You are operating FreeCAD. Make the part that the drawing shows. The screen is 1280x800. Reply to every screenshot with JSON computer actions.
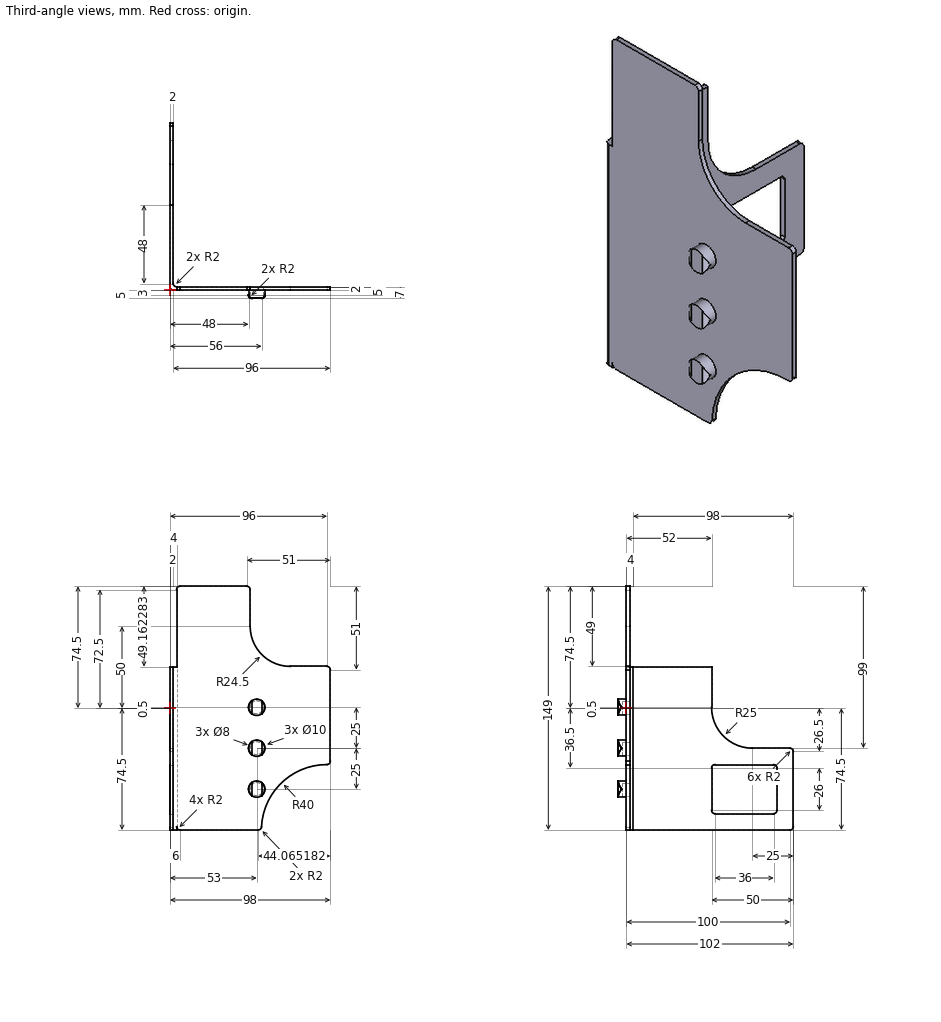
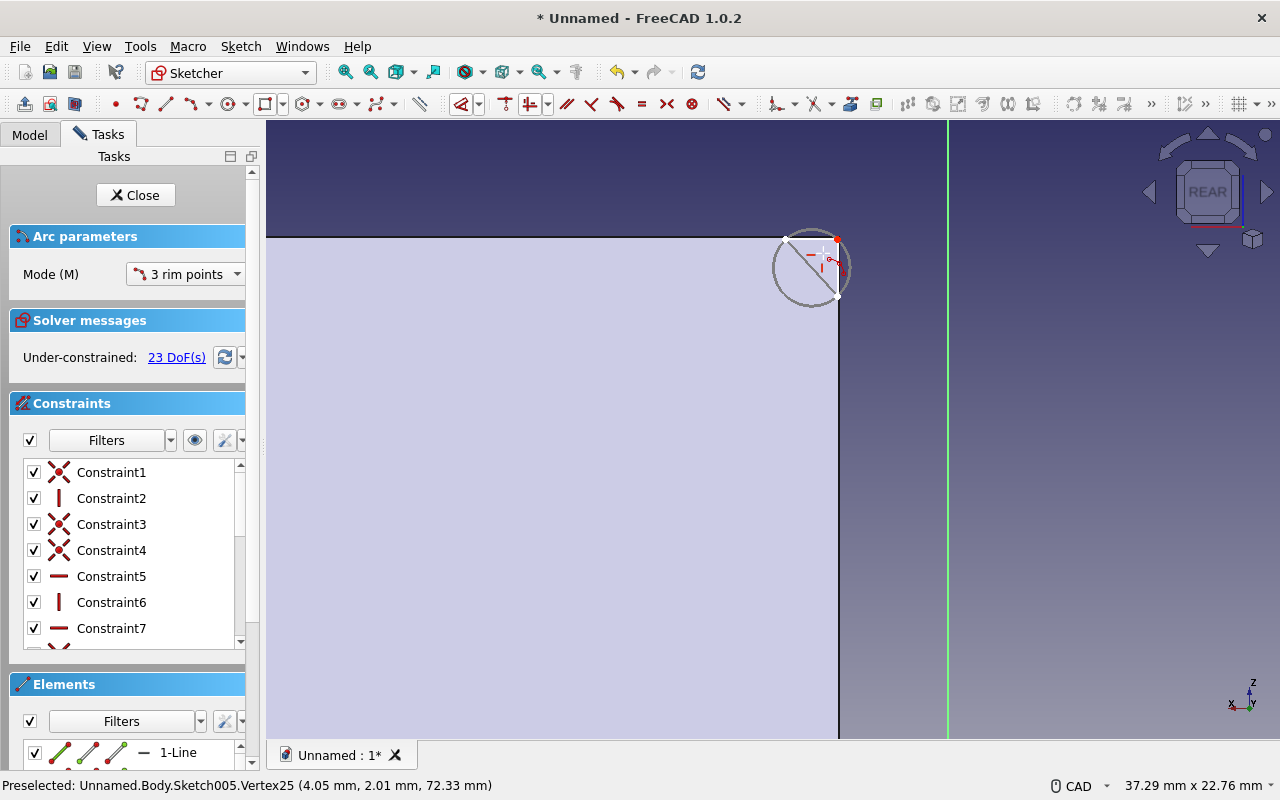
{"action": "left_click", "coordinate": [823, 253]}
{"action": "key", "text": "Escape"}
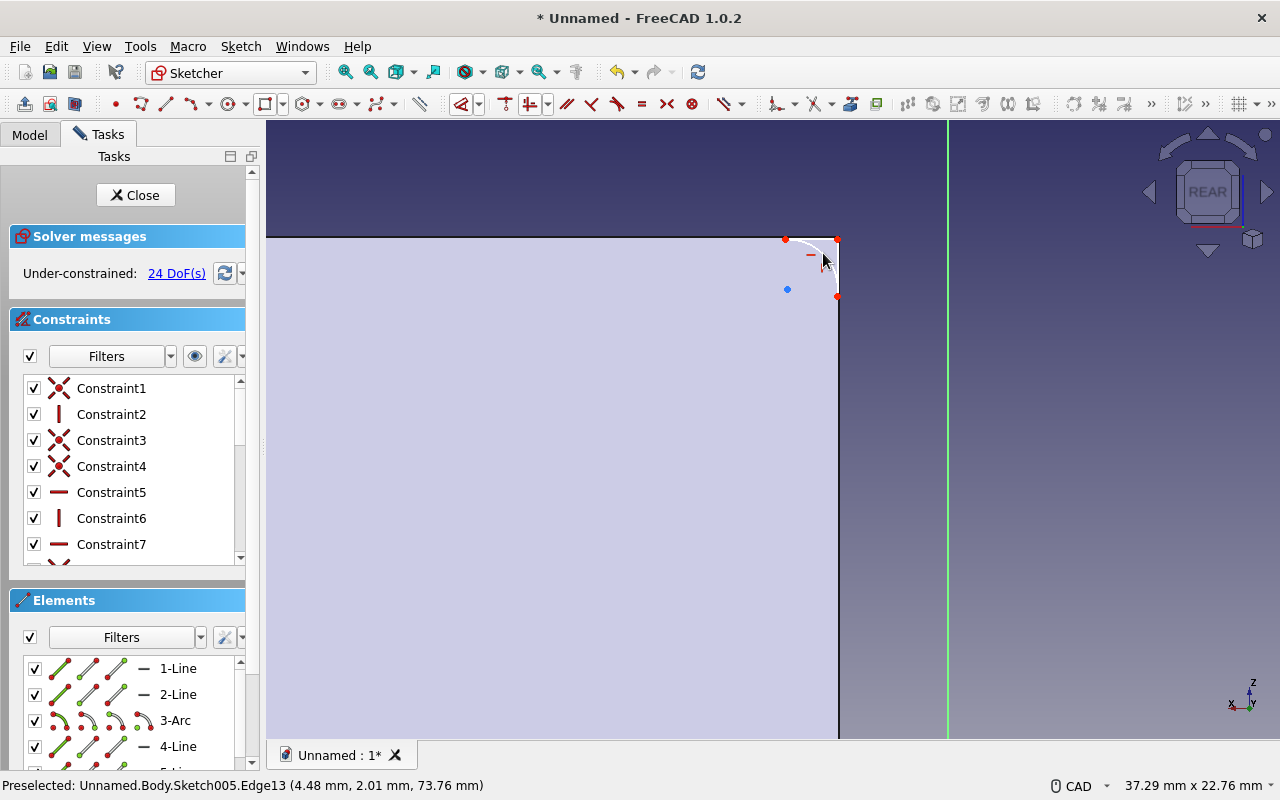
{"action": "scroll", "coordinate": [813, 247], "scroll_direction": "down", "scroll_amount": 12}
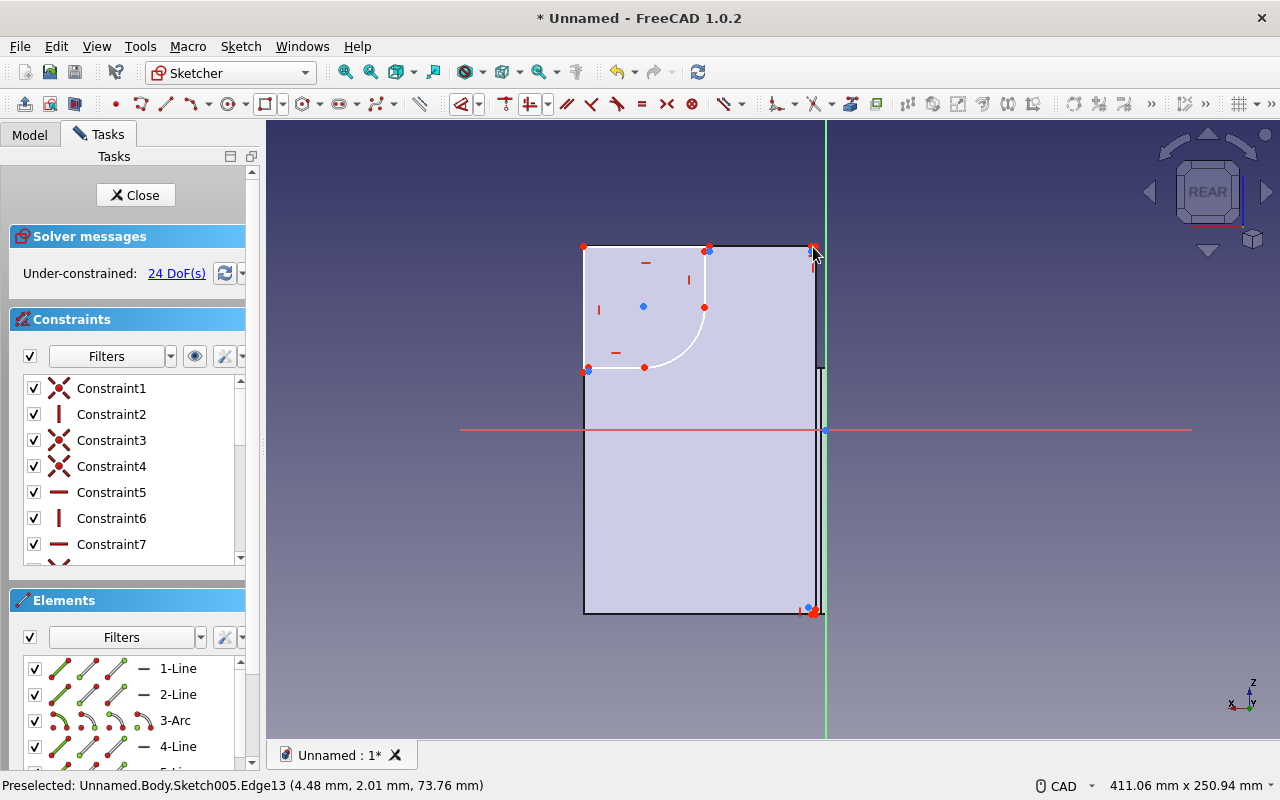
{"action": "scroll", "coordinate": [815, 614], "scroll_direction": "up", "scroll_amount": 12}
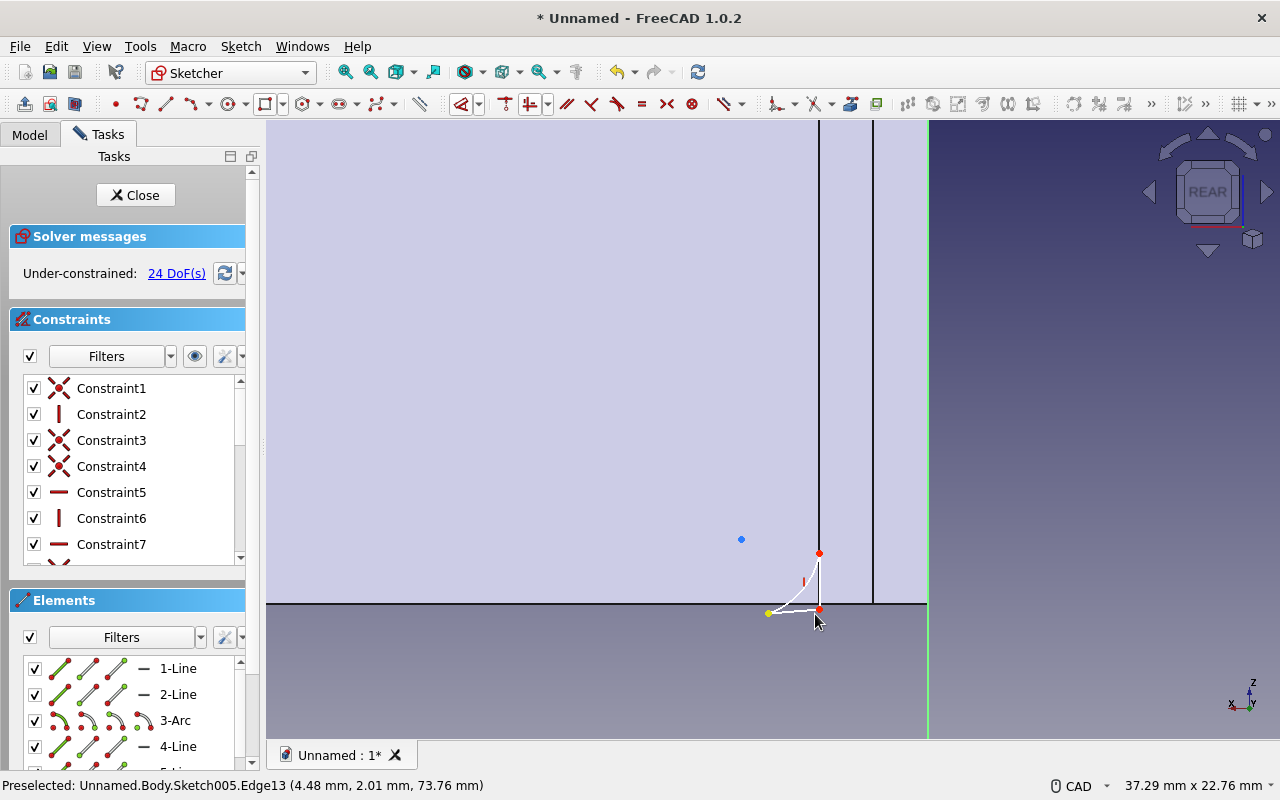
{"action": "left_click", "coordinate": [804, 611]}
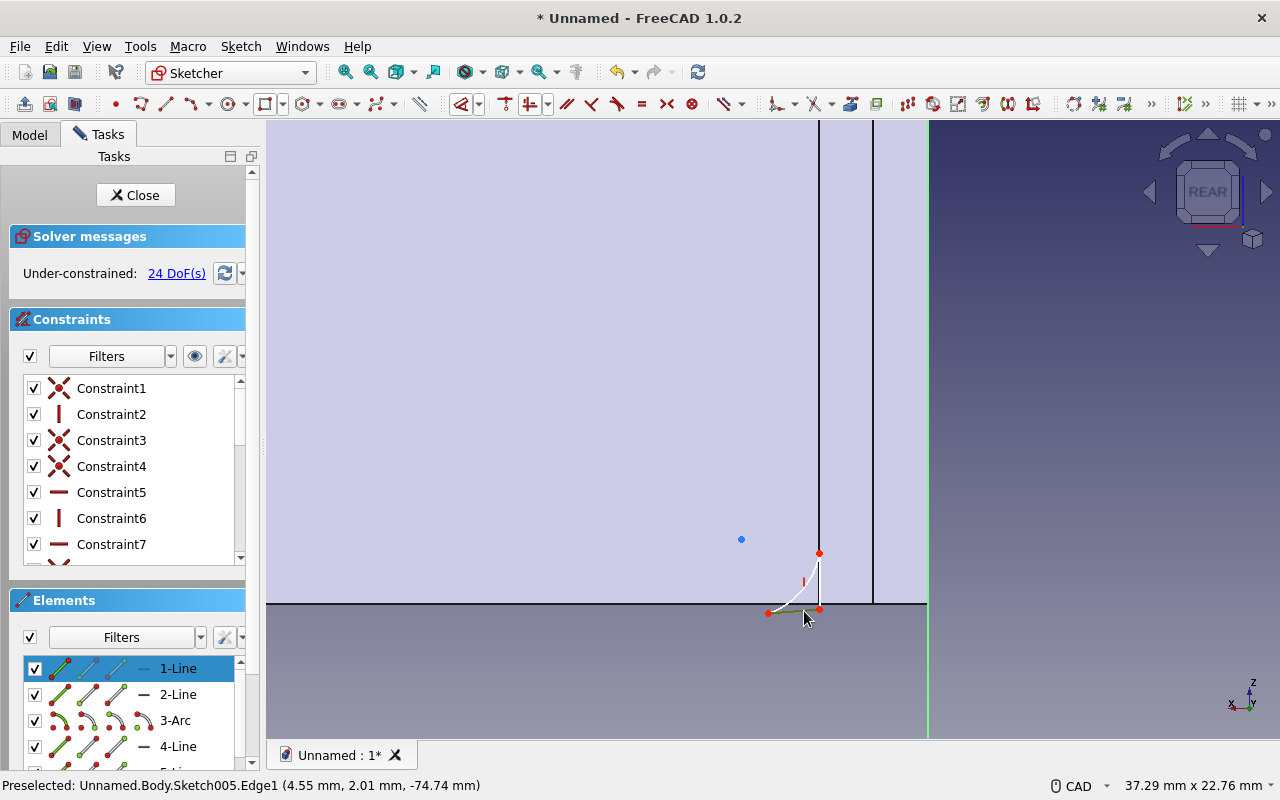
{"action": "scroll", "coordinate": [790, 602], "scroll_direction": "up", "scroll_amount": 2}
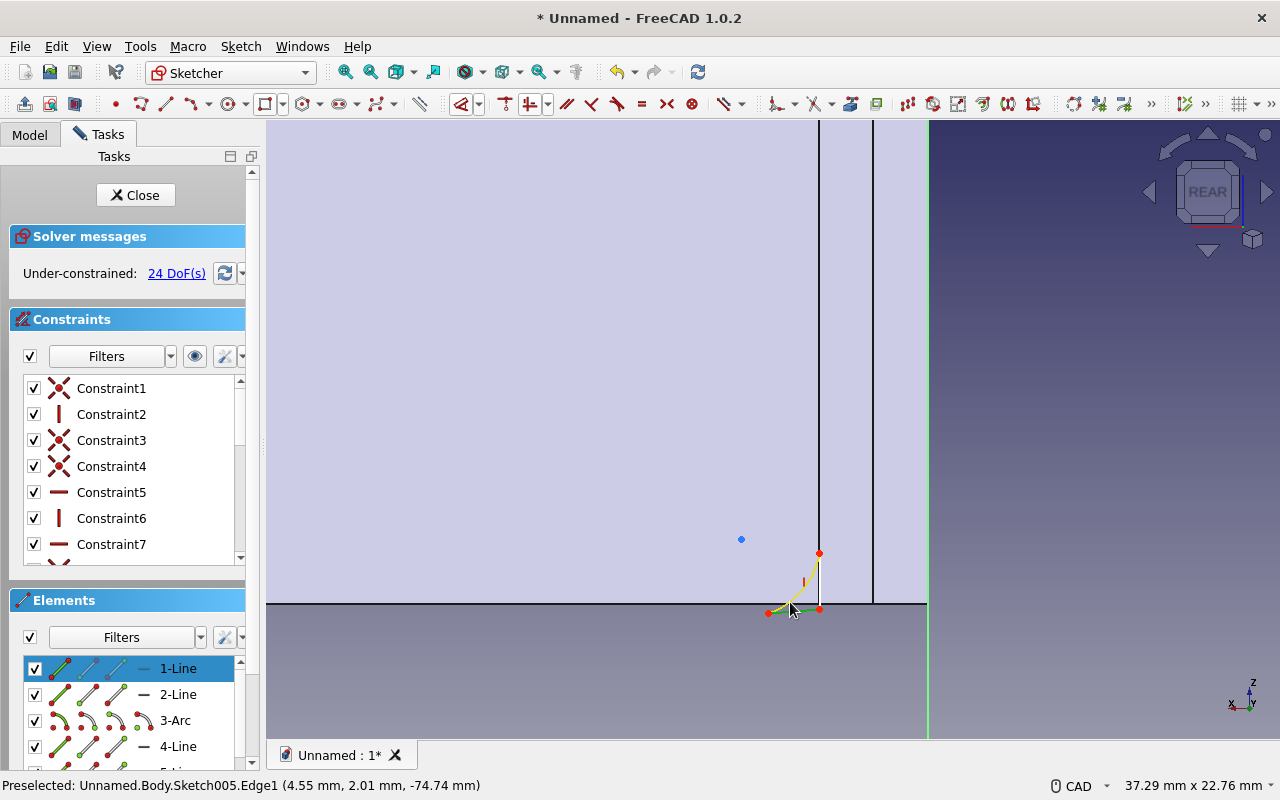
{"action": "left_click", "coordinate": [790, 601]}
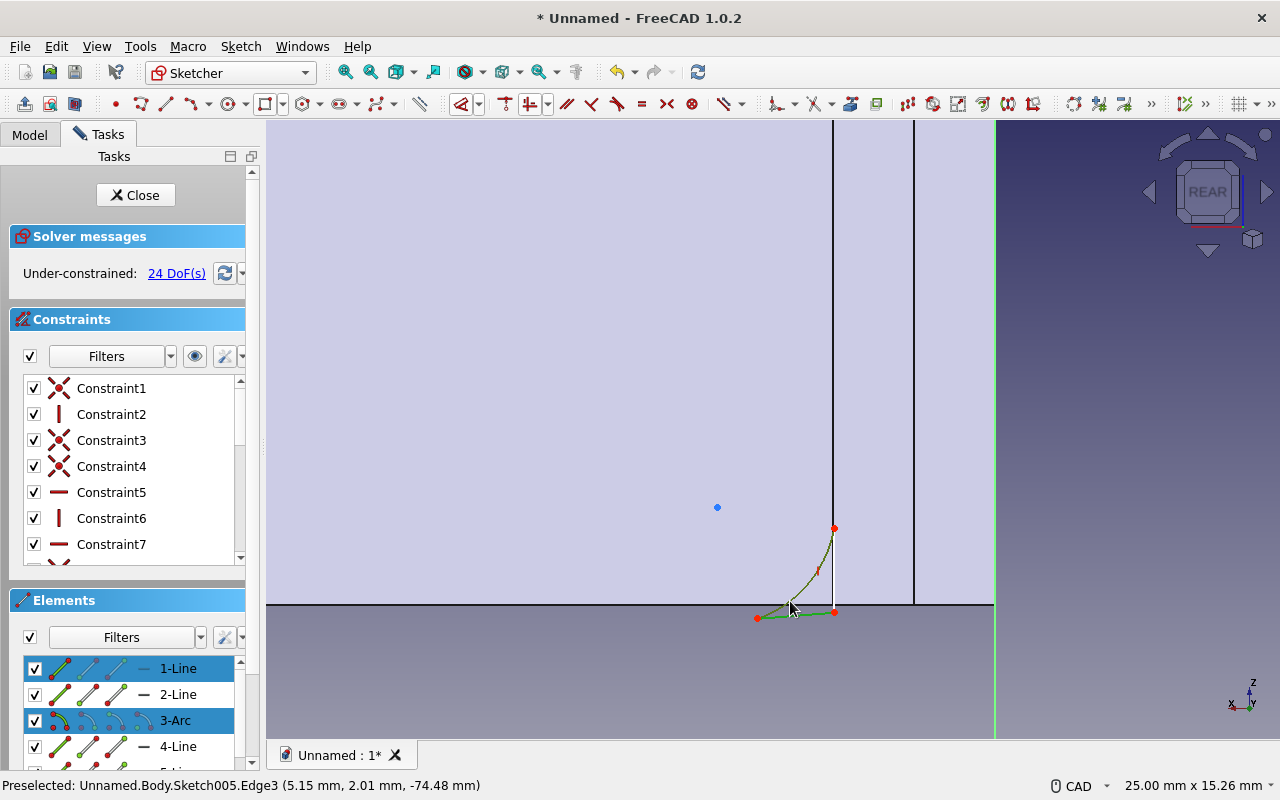
{"action": "key", "text": "t"}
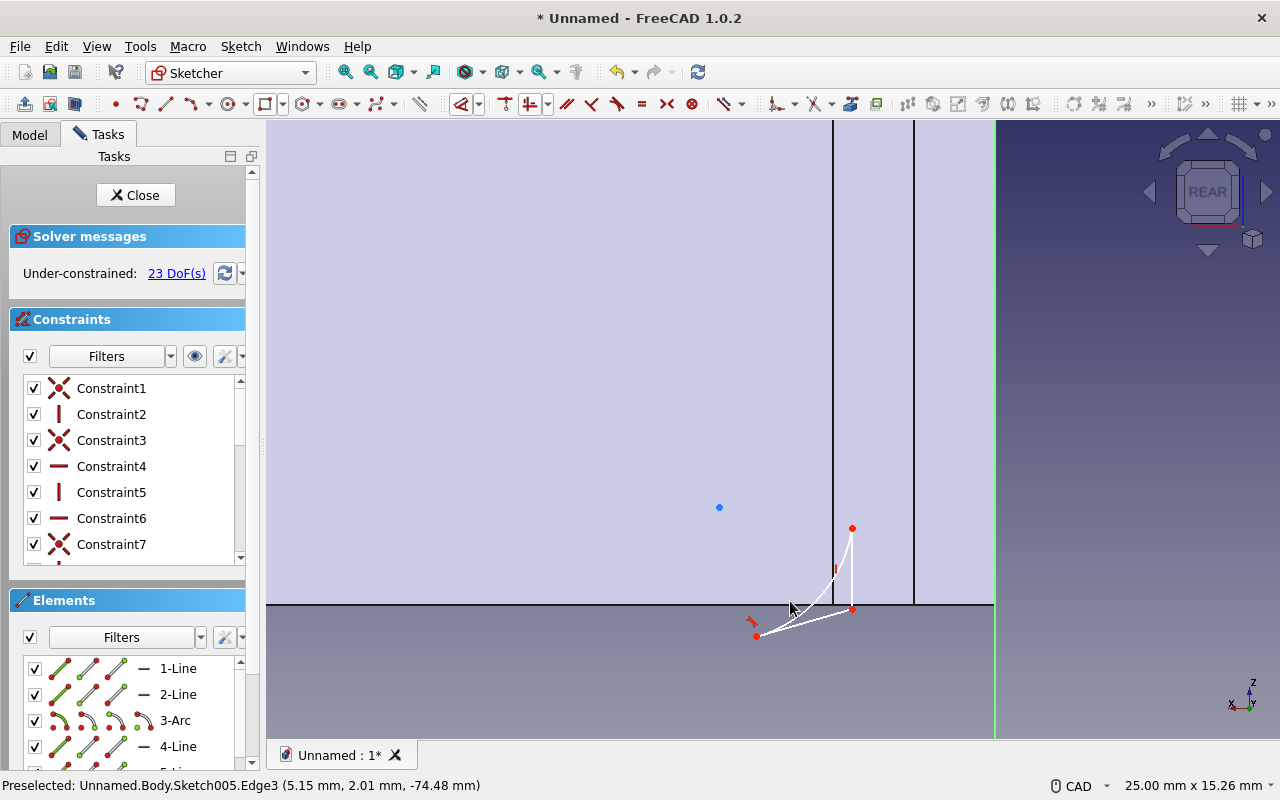
{"action": "left_click", "coordinate": [852, 585]}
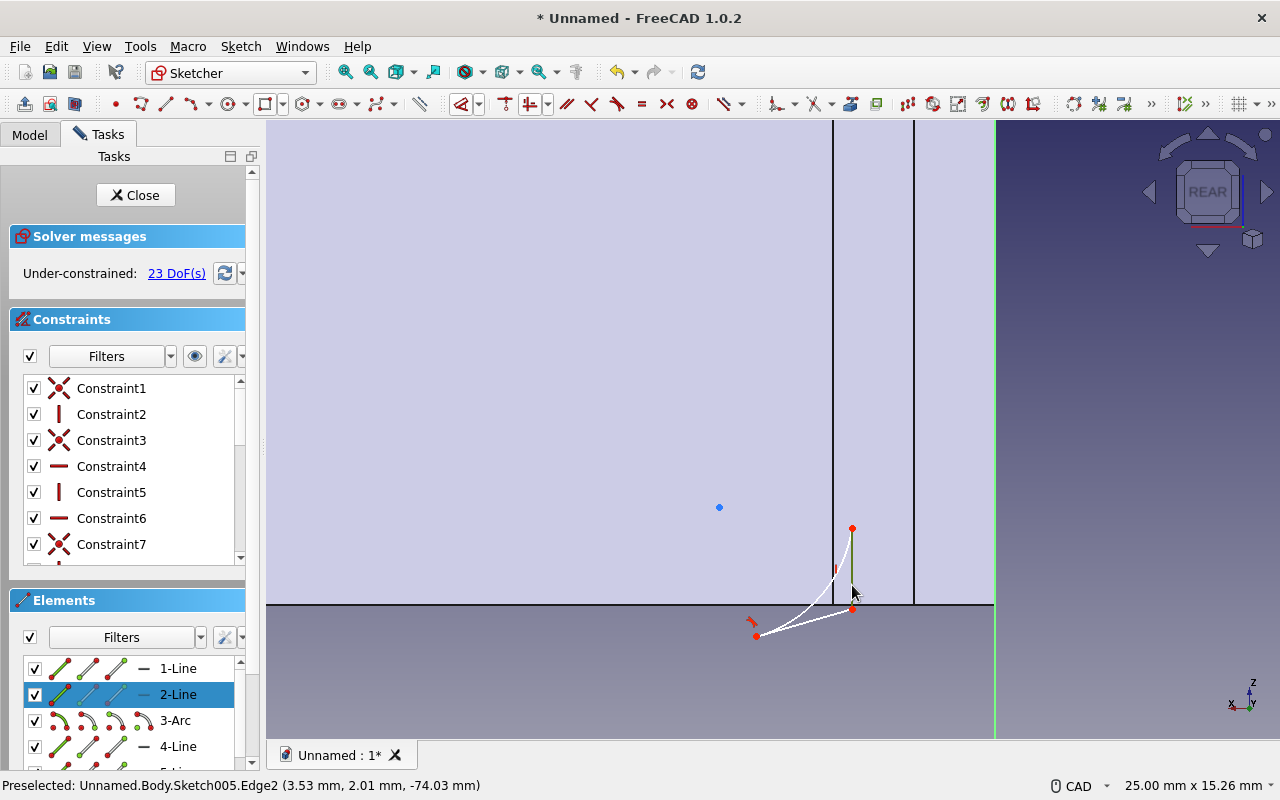
{"action": "left_click", "coordinate": [820, 597]}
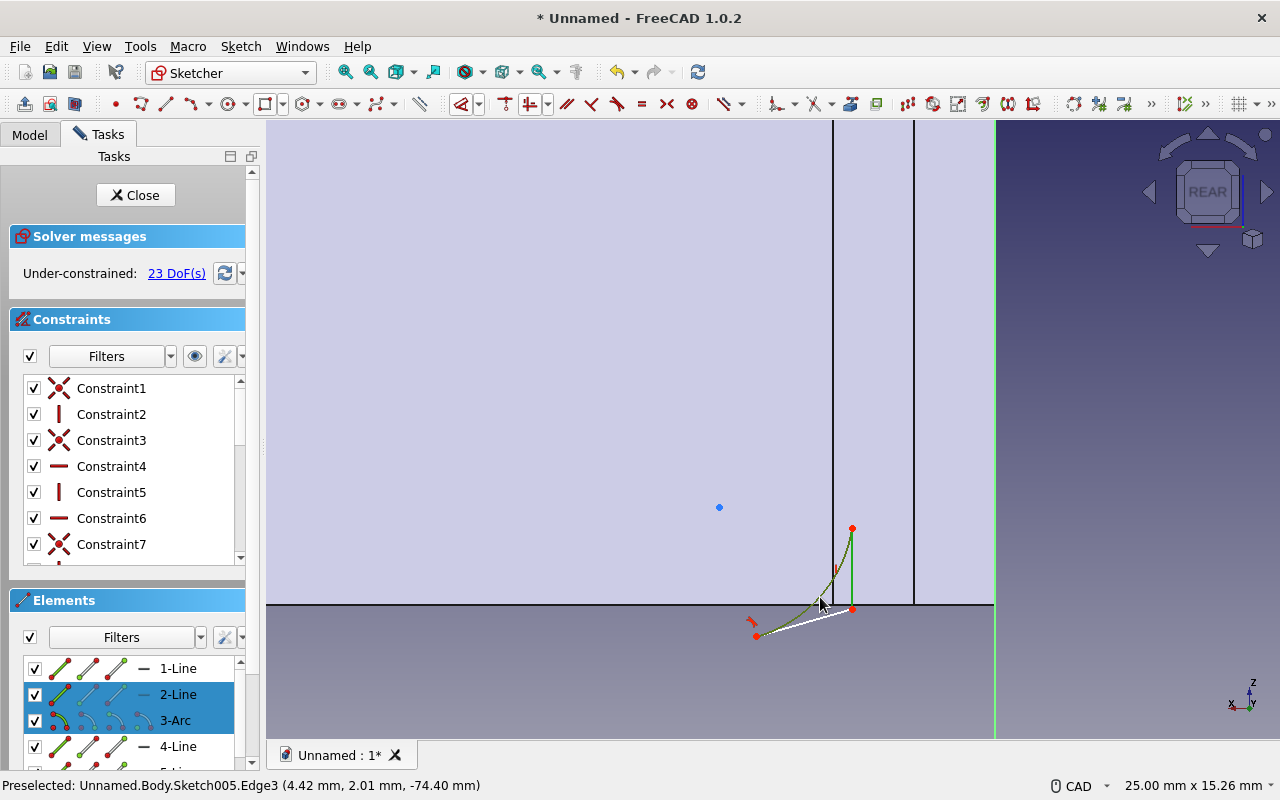
{"action": "key", "text": "t"}